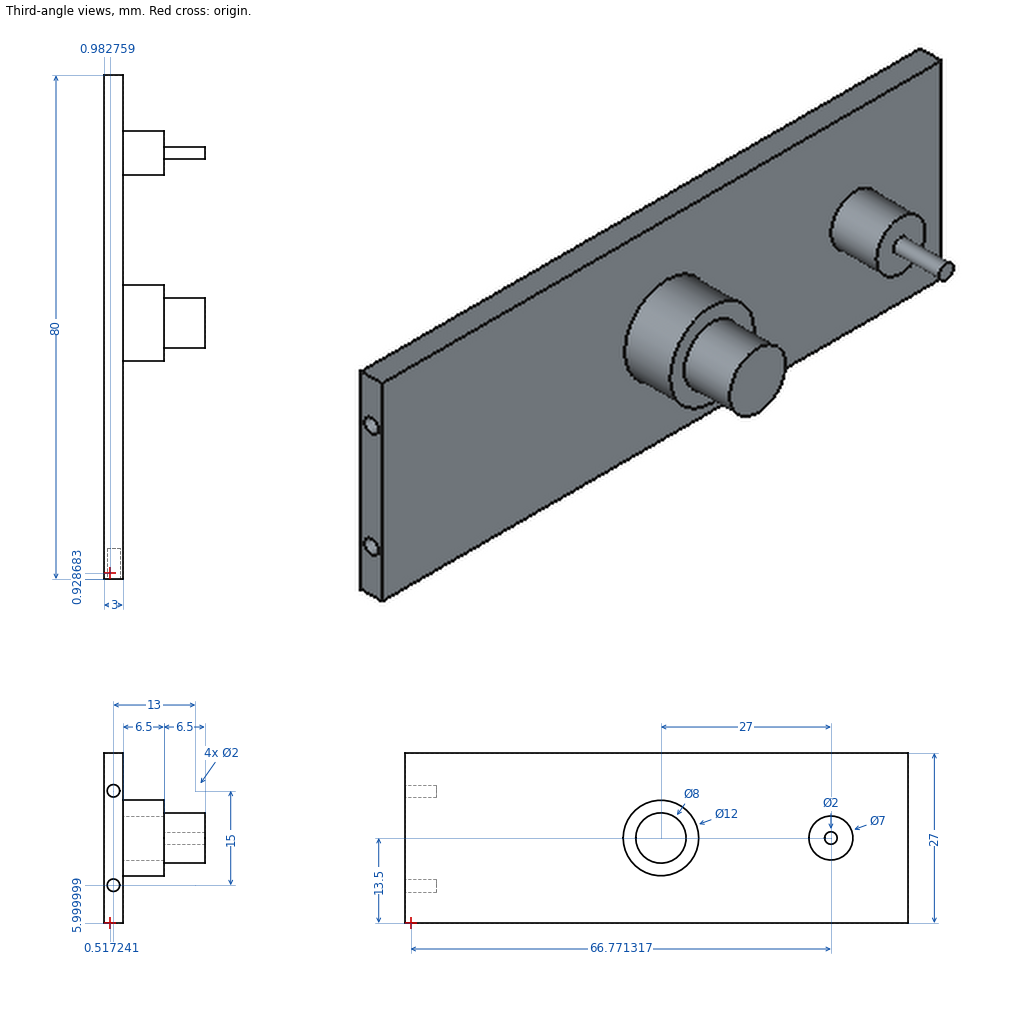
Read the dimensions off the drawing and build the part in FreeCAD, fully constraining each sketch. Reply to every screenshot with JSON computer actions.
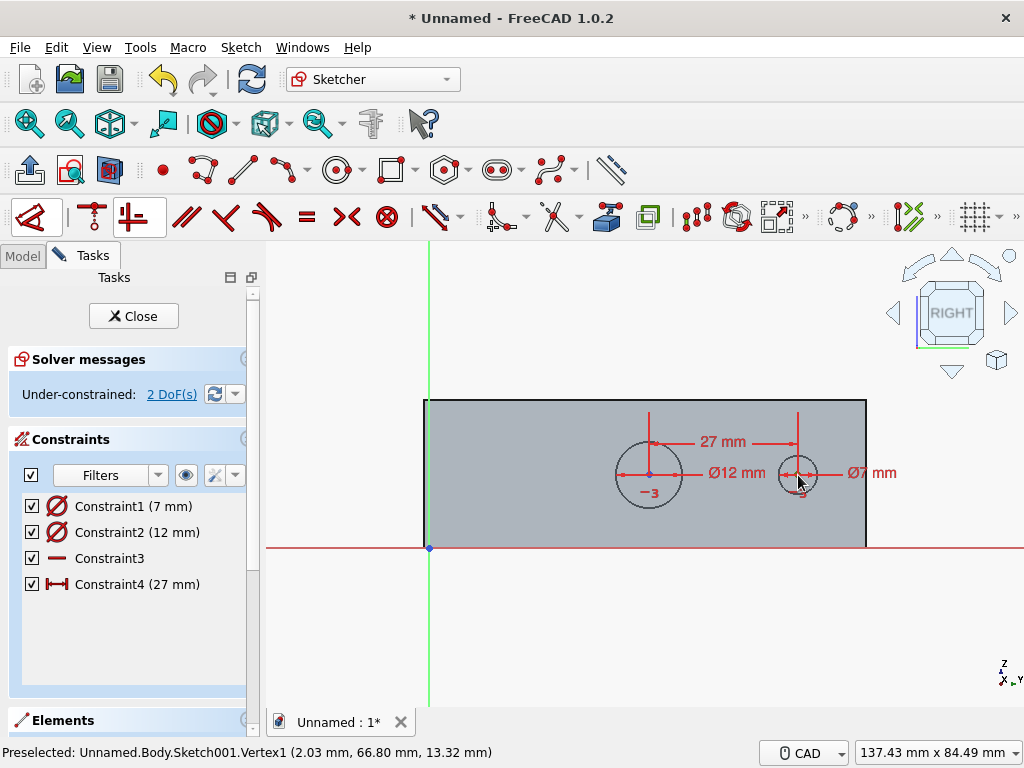
{"action": "left_click", "coordinate": [56, 218]}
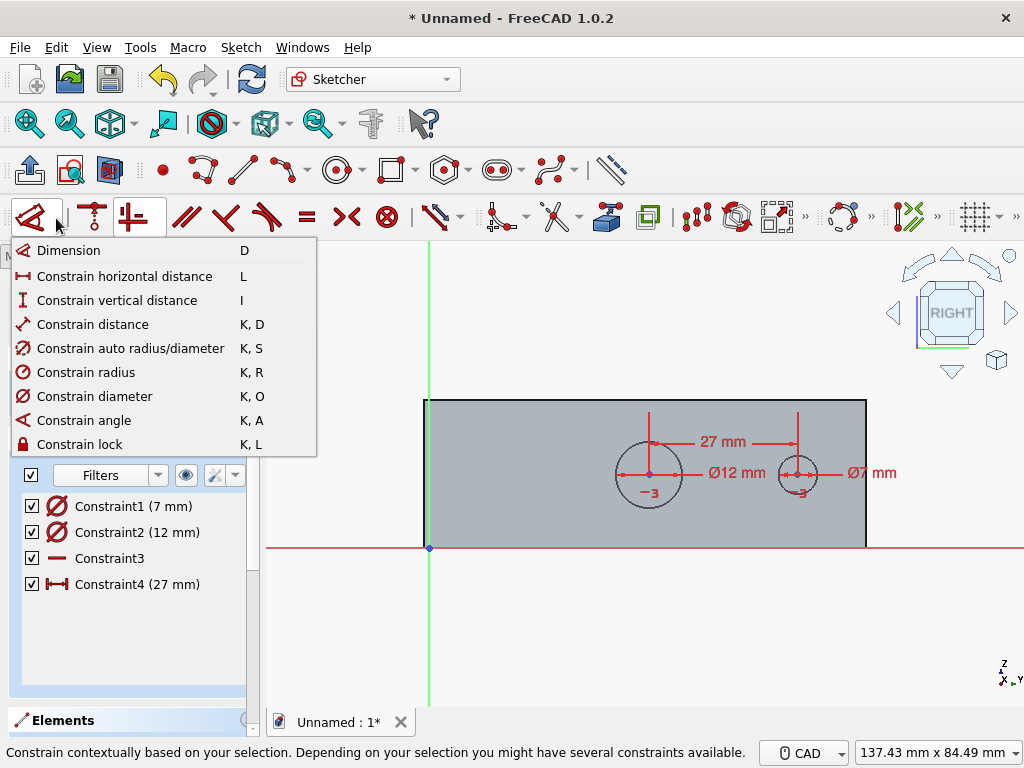
{"action": "left_click", "coordinate": [164, 300]}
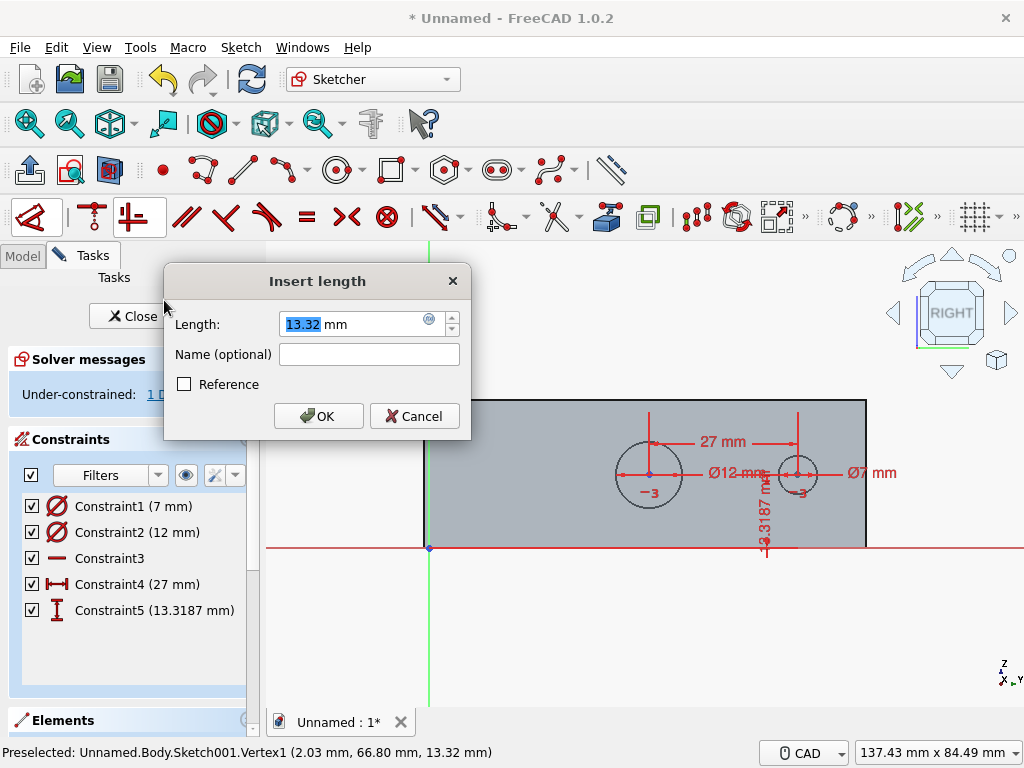
{"action": "type", "text": "13.5"}
{"action": "key", "text": "Return"}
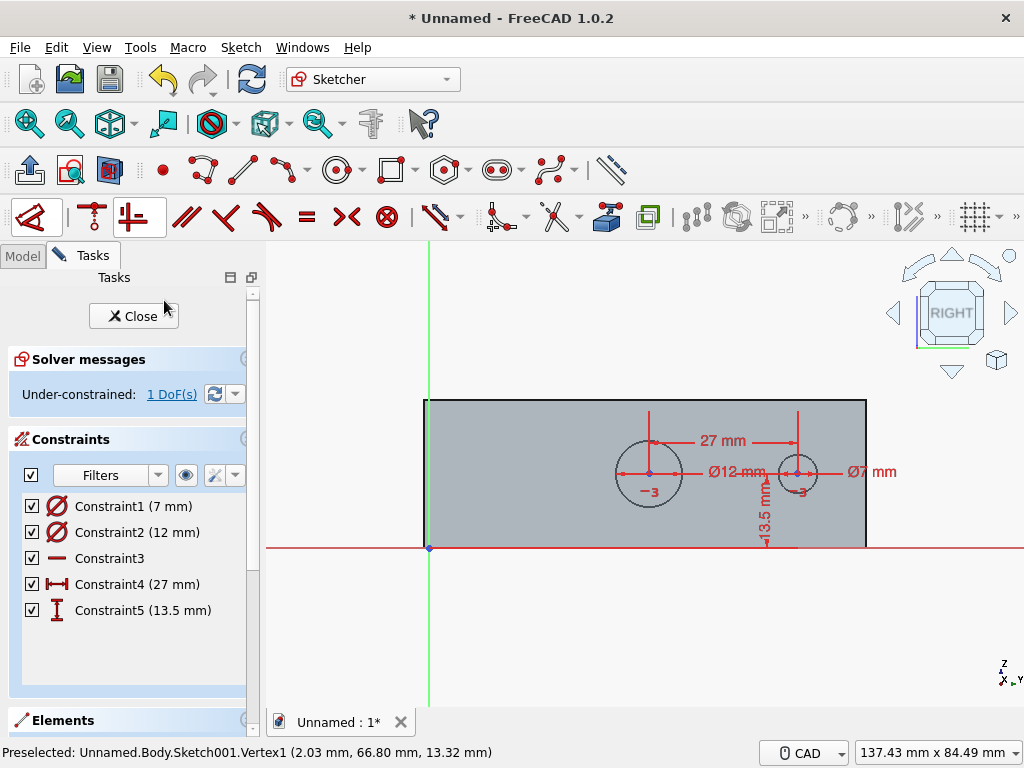
{"action": "left_click", "coordinate": [798, 474]}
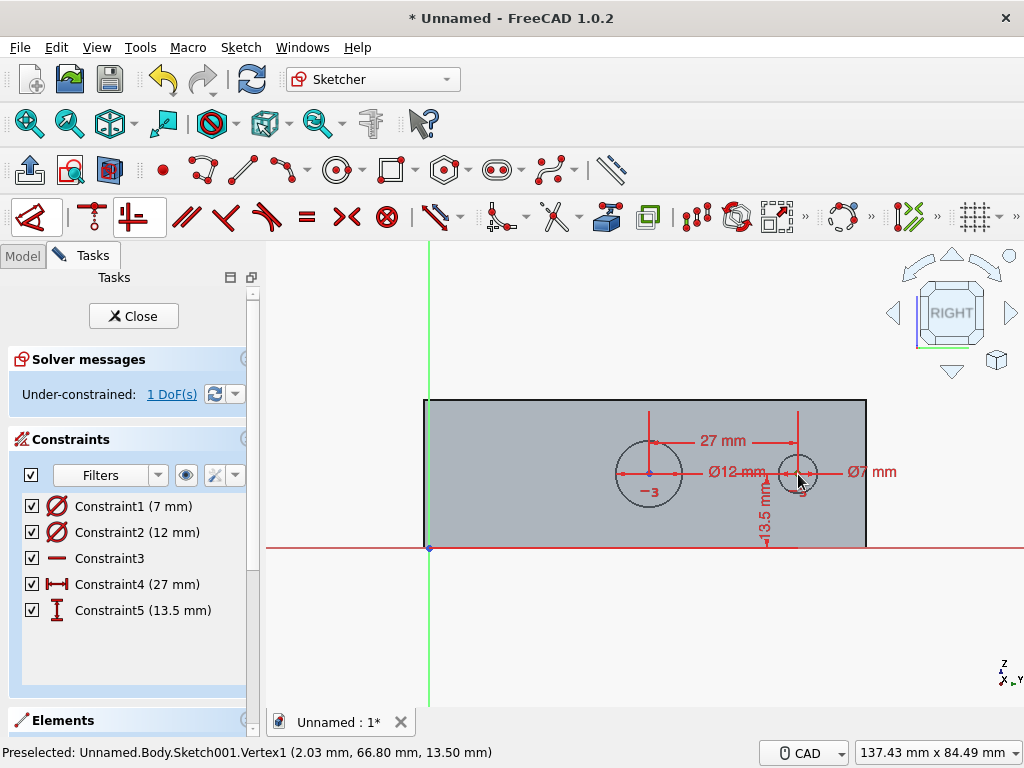
{"action": "key", "text": "l"}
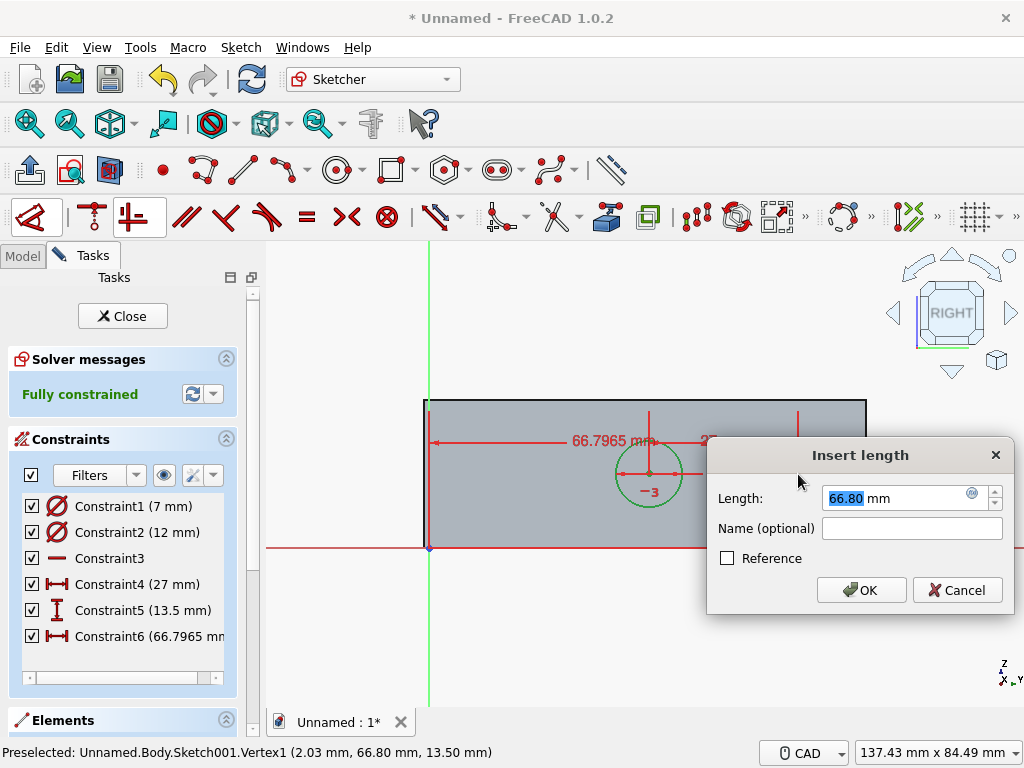
{"action": "type", "text": "66.771317"}
{"action": "key", "text": "Return"}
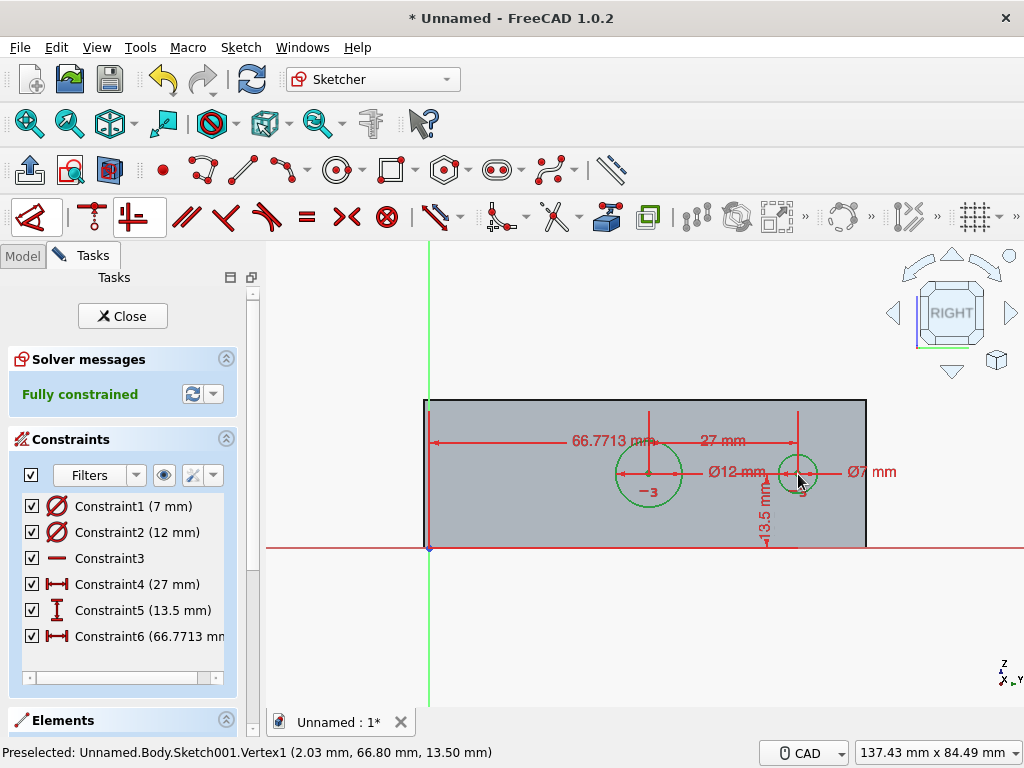
{"action": "left_click", "coordinate": [123, 316]}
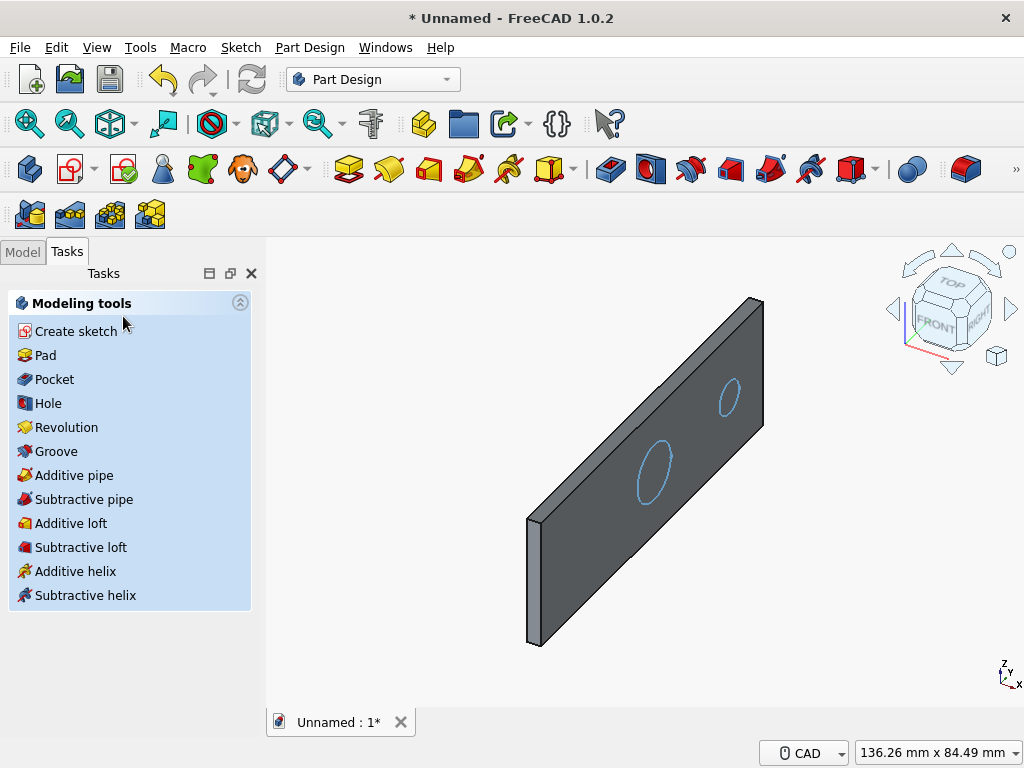
{"action": "left_click", "coordinate": [350, 170]}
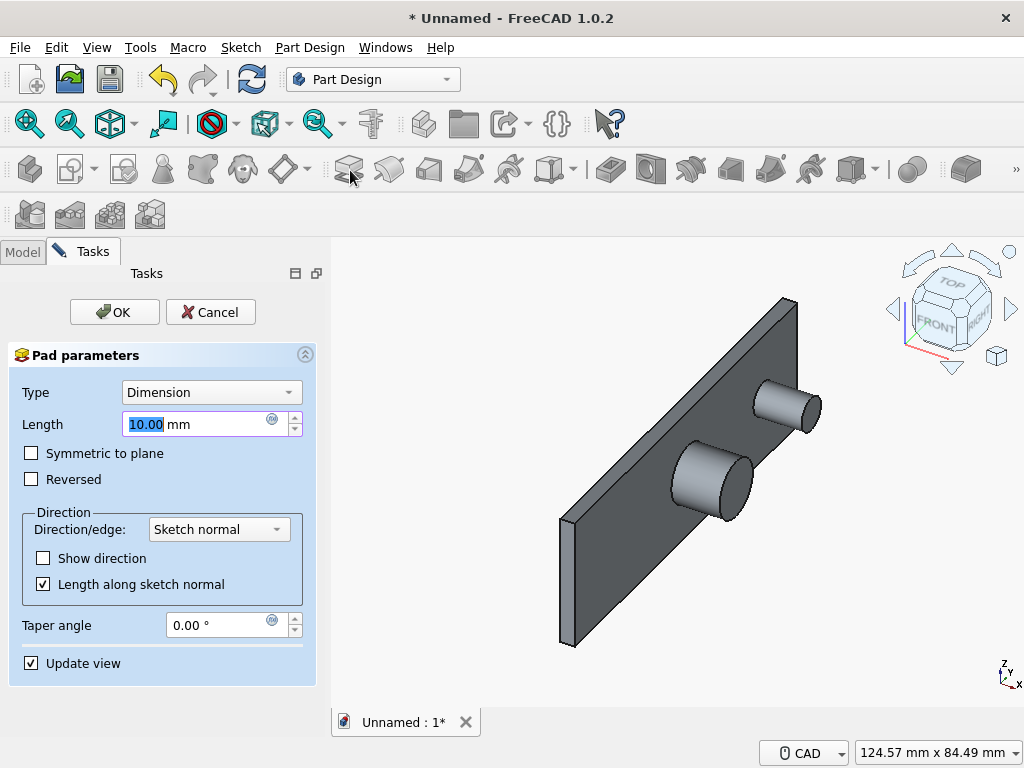
{"action": "type", "text": "6.5"}
{"action": "key", "text": "Tab"}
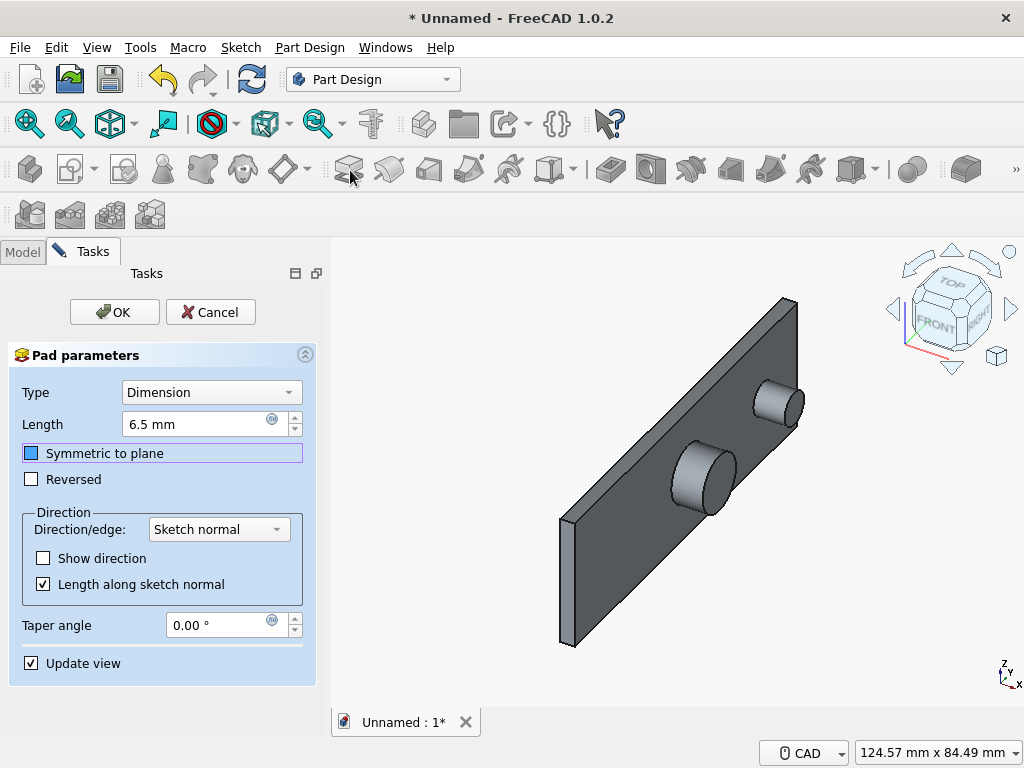
{"action": "left_click", "coordinate": [115, 312]}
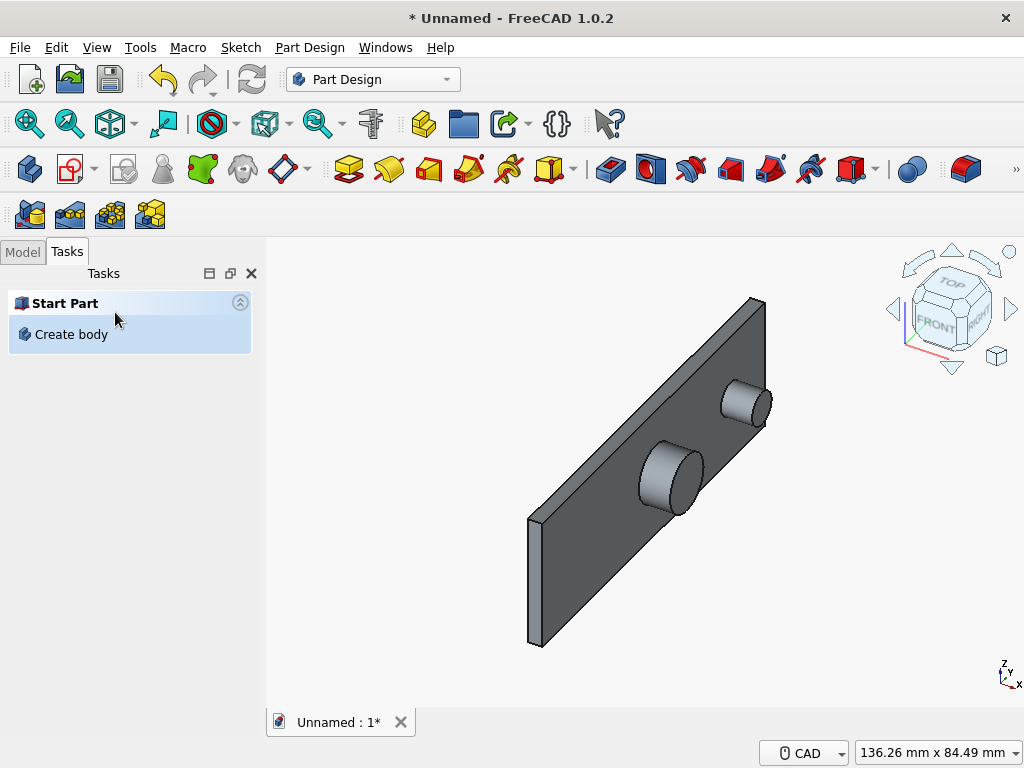
{"action": "left_click", "coordinate": [687, 482]}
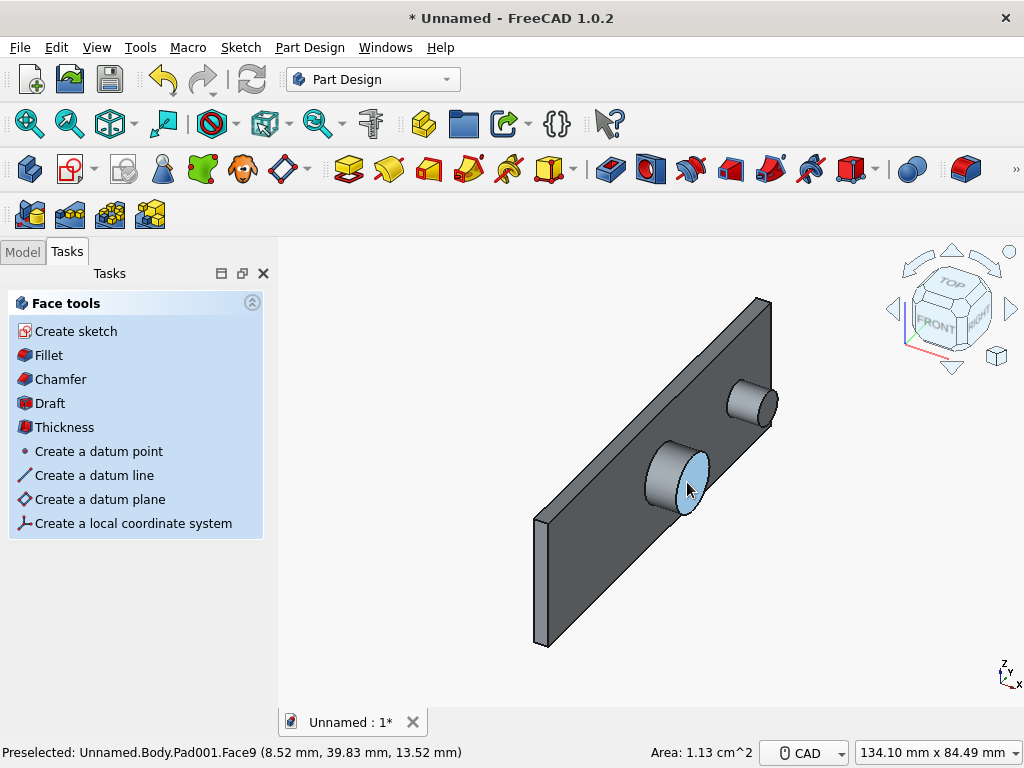
{"action": "left_click", "coordinate": [70, 170]}